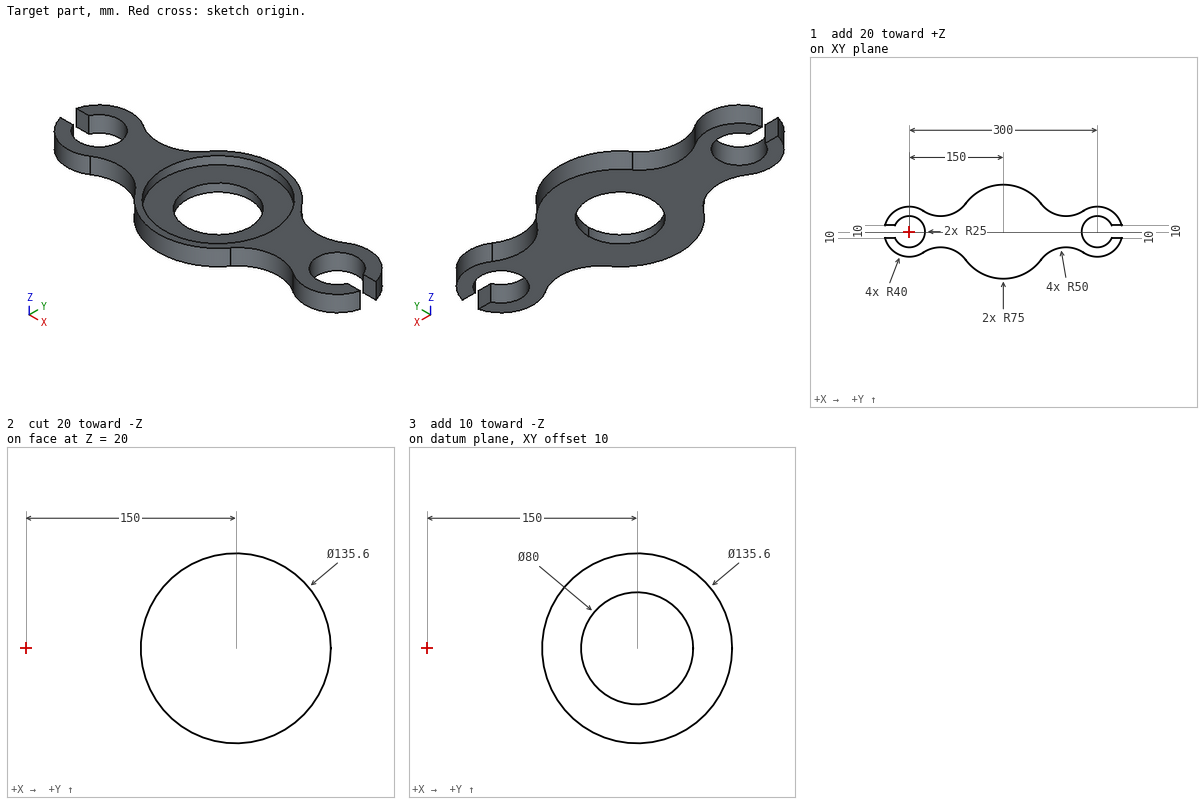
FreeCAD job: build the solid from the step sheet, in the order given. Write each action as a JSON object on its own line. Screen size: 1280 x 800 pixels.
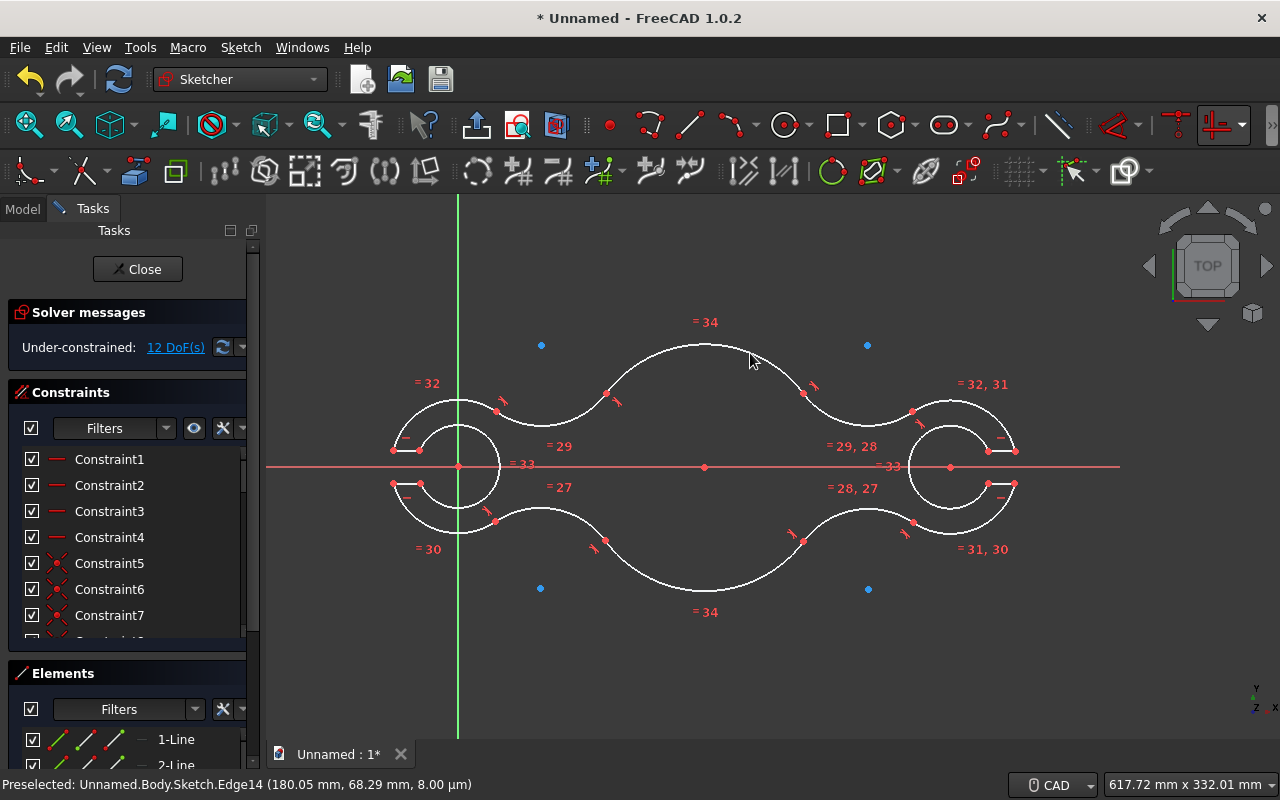
{"action": "left_click", "coordinate": [705, 468]}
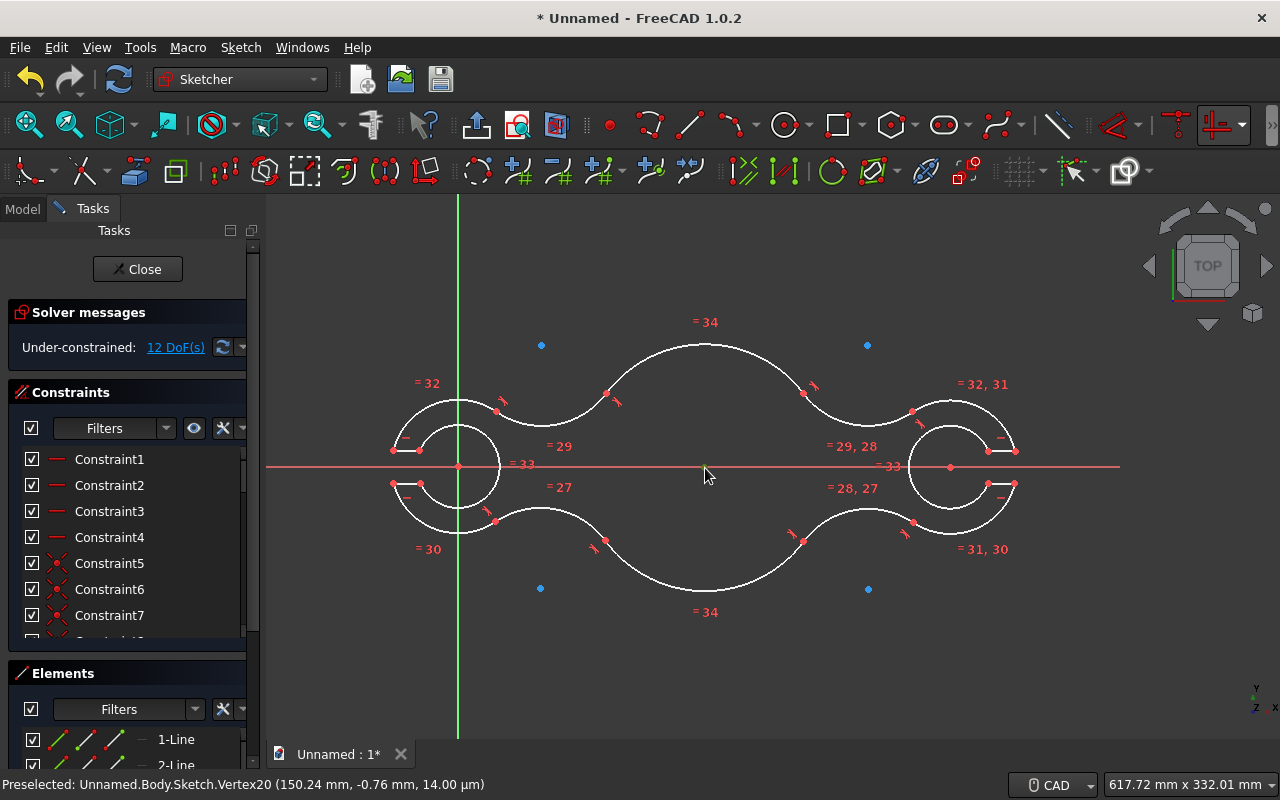
{"action": "left_click", "coordinate": [353, 466]}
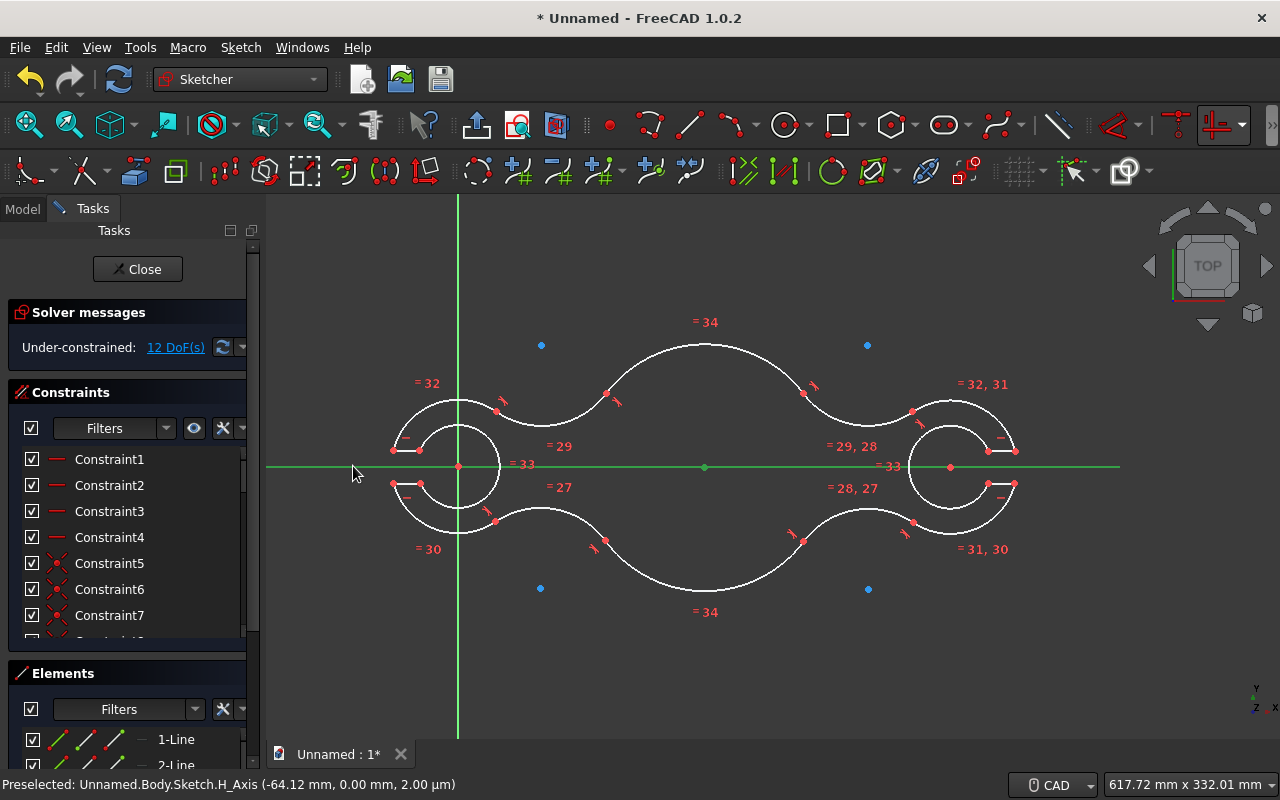
{"action": "left_click", "coordinate": [1176, 126]}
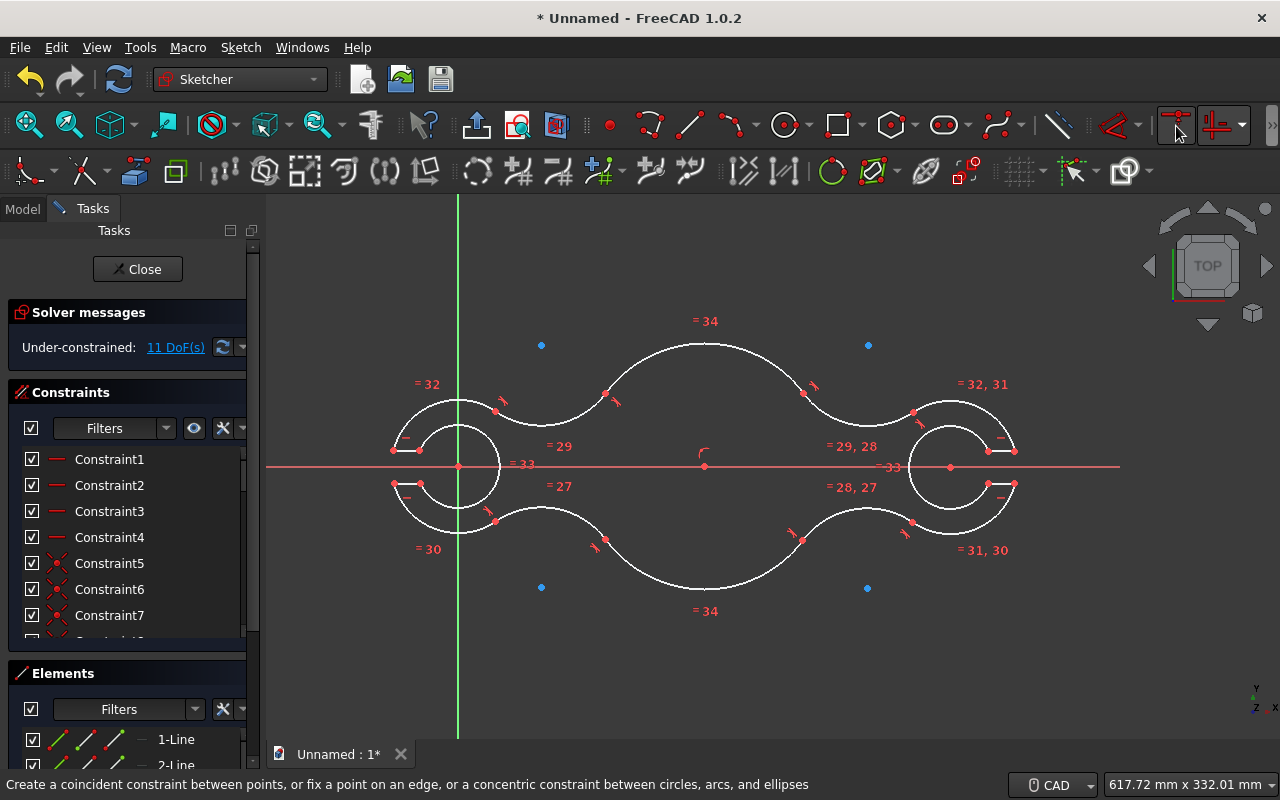
{"action": "left_click", "coordinate": [950, 468]}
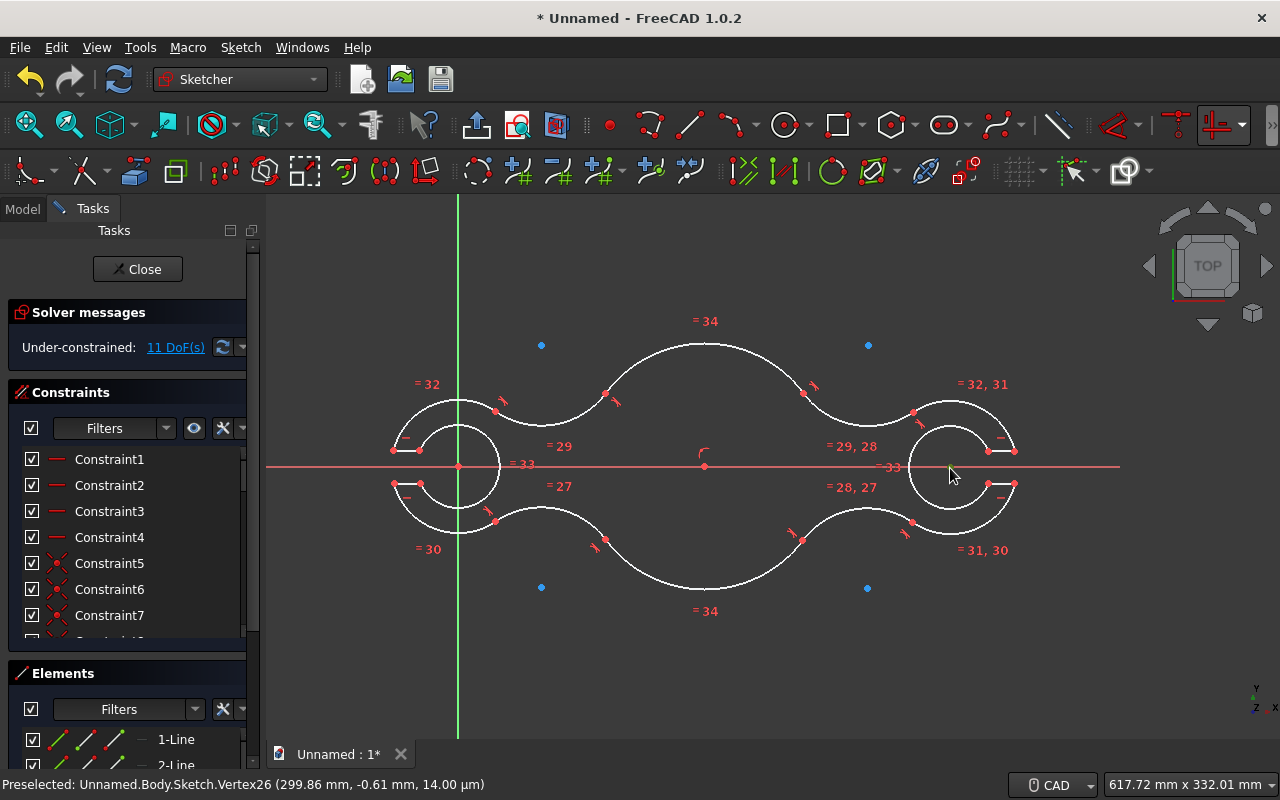
{"action": "left_click", "coordinate": [353, 466]}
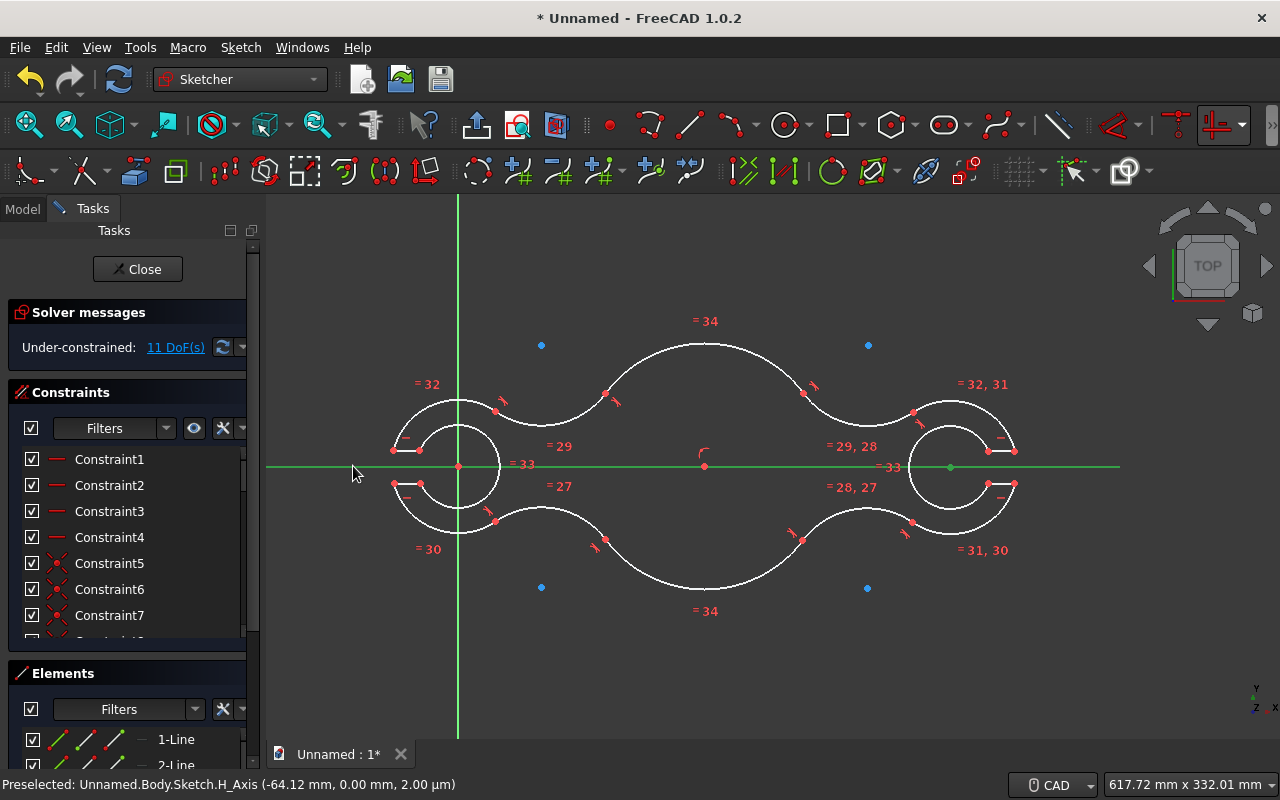
{"action": "left_click", "coordinate": [1176, 126]}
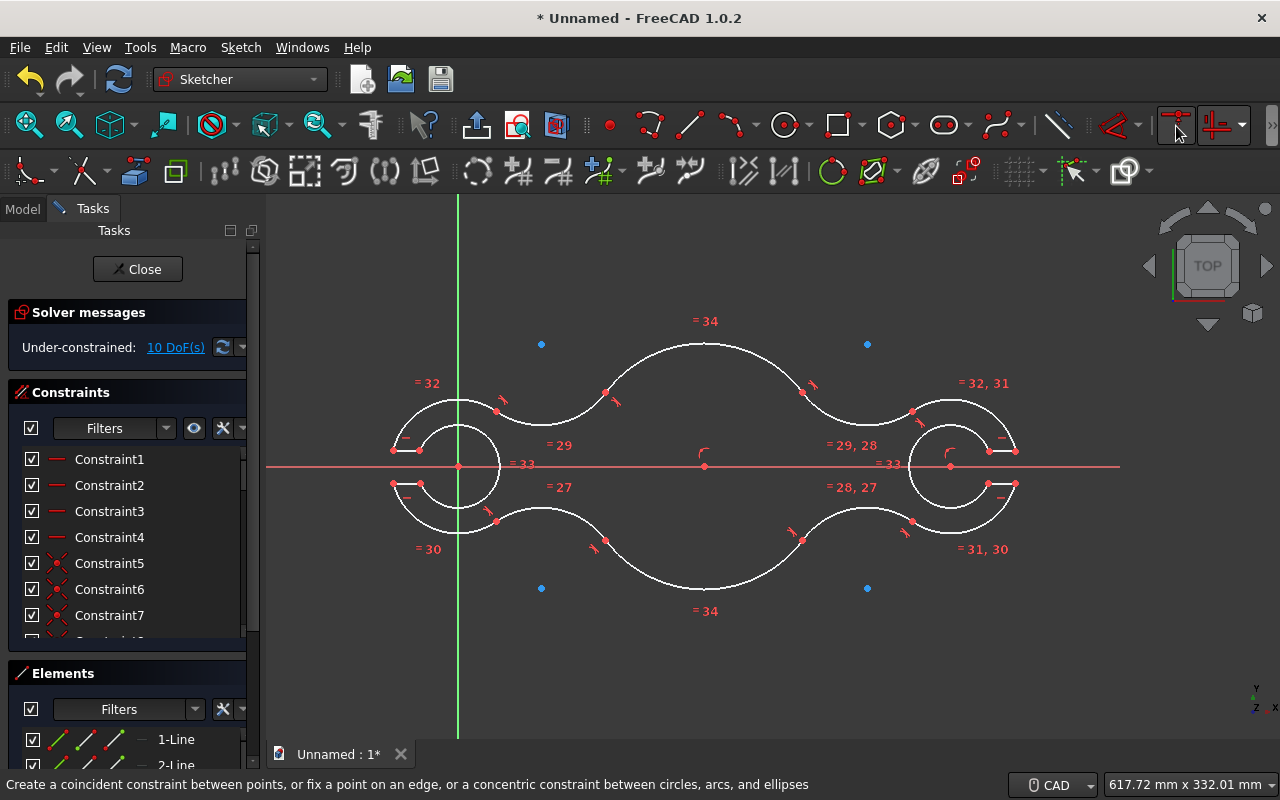
{"action": "left_click", "coordinate": [478, 503]}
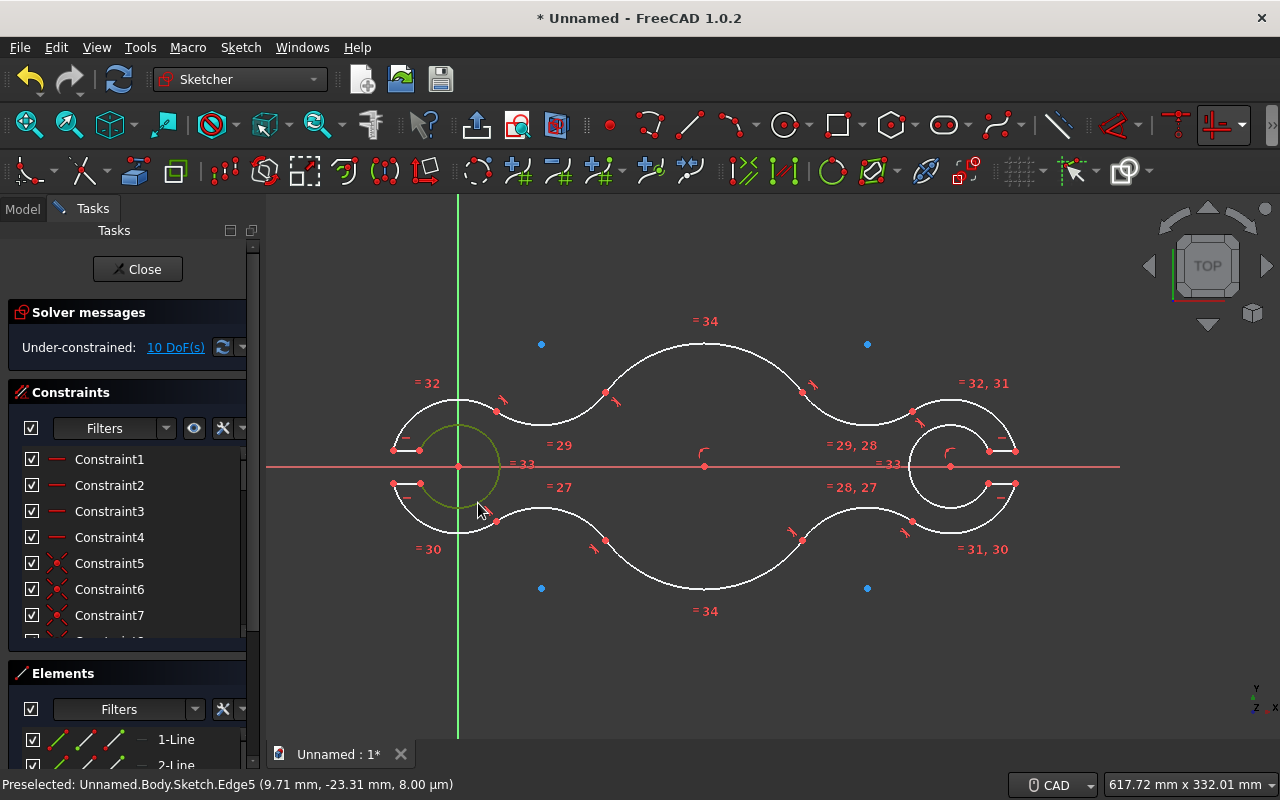
{"action": "key", "text": "k r"}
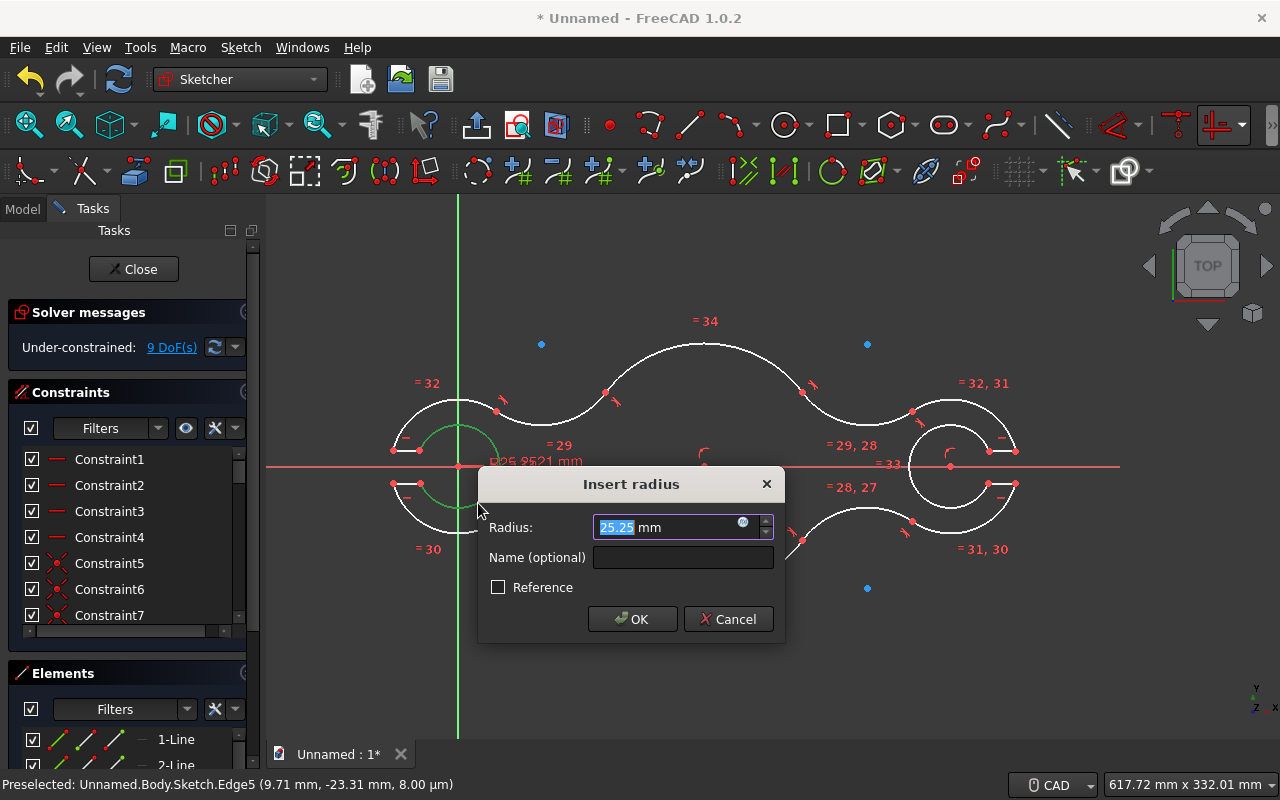
{"action": "type", "text": "25"}
{"action": "key", "text": "Return"}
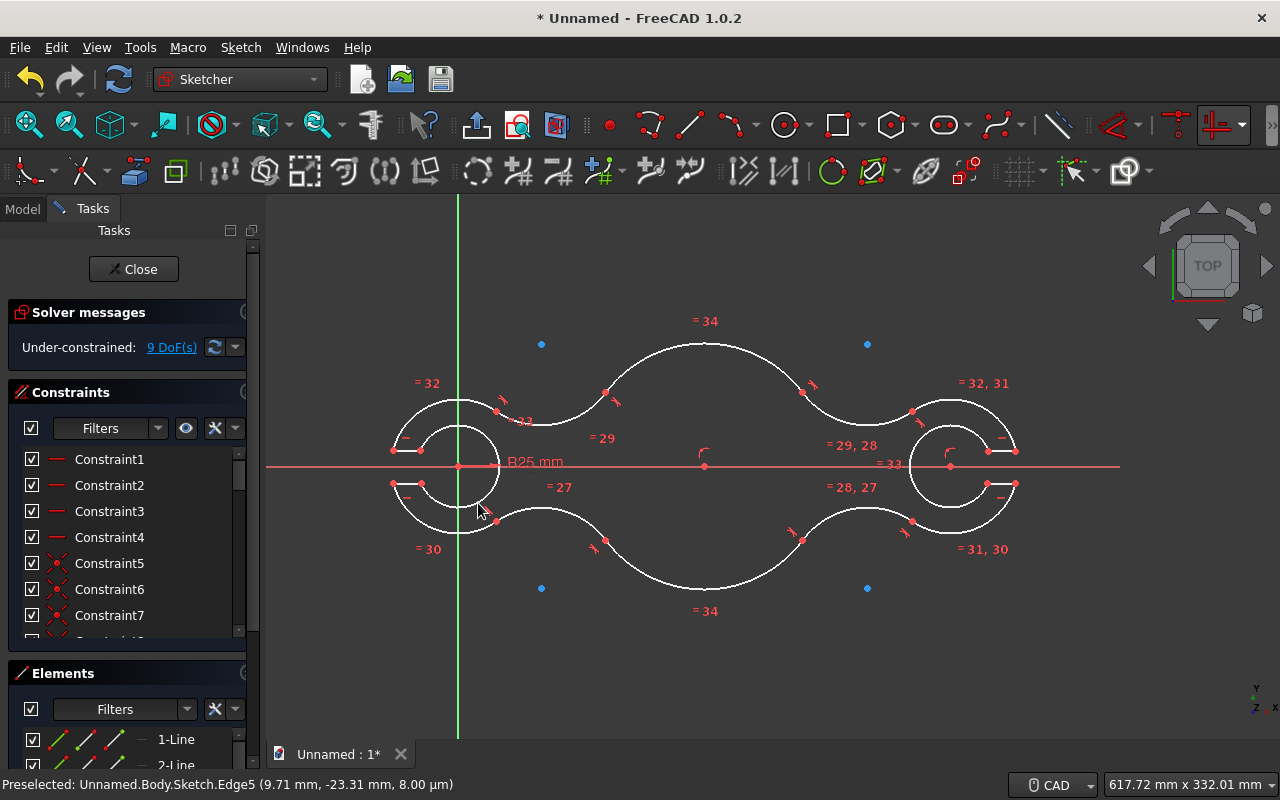
{"action": "left_click", "coordinate": [413, 516]}